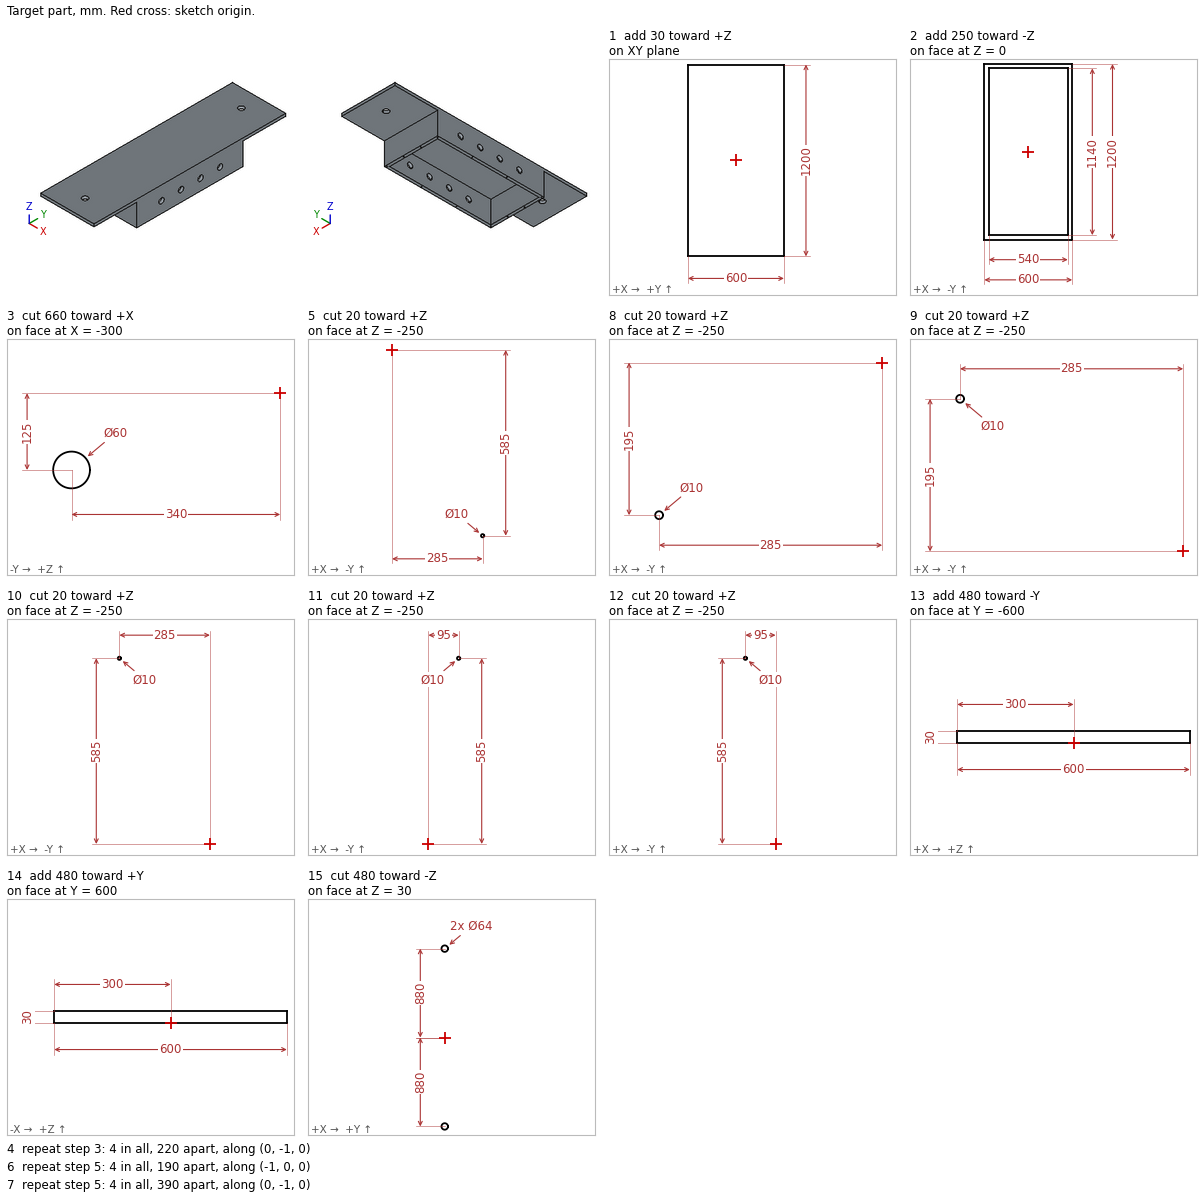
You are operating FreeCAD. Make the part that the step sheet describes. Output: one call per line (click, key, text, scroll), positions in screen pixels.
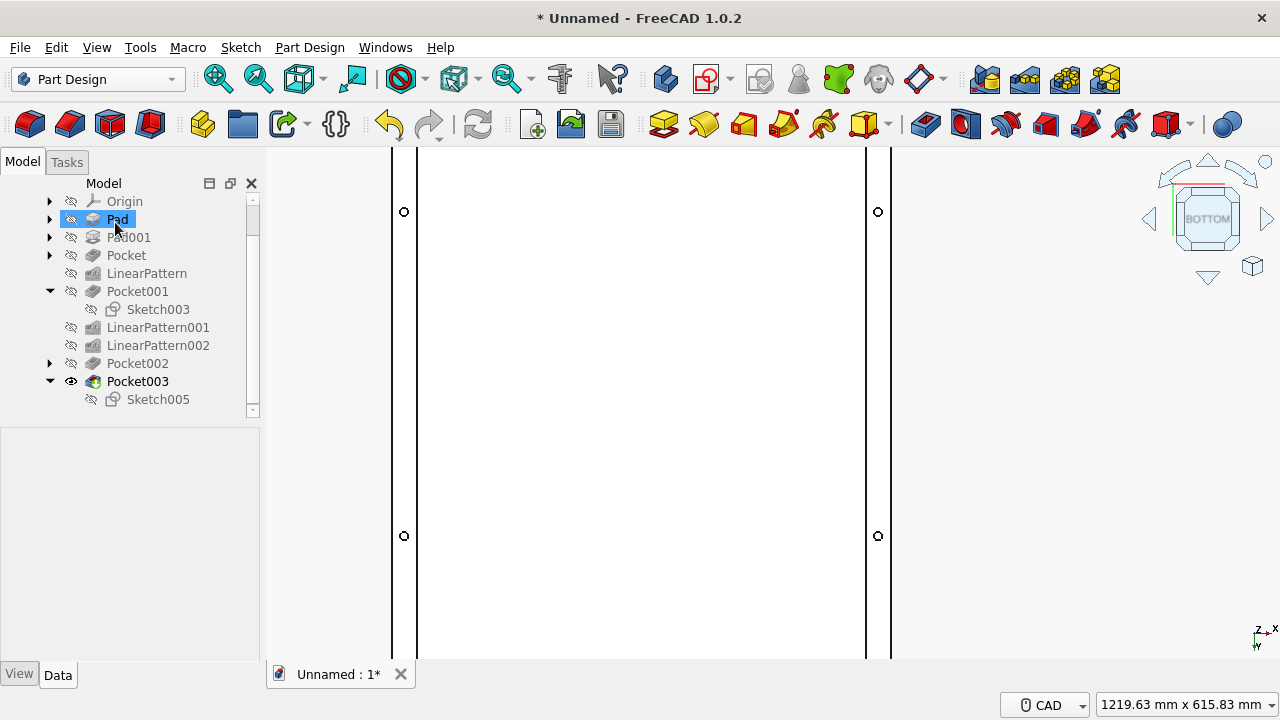
click(220, 80)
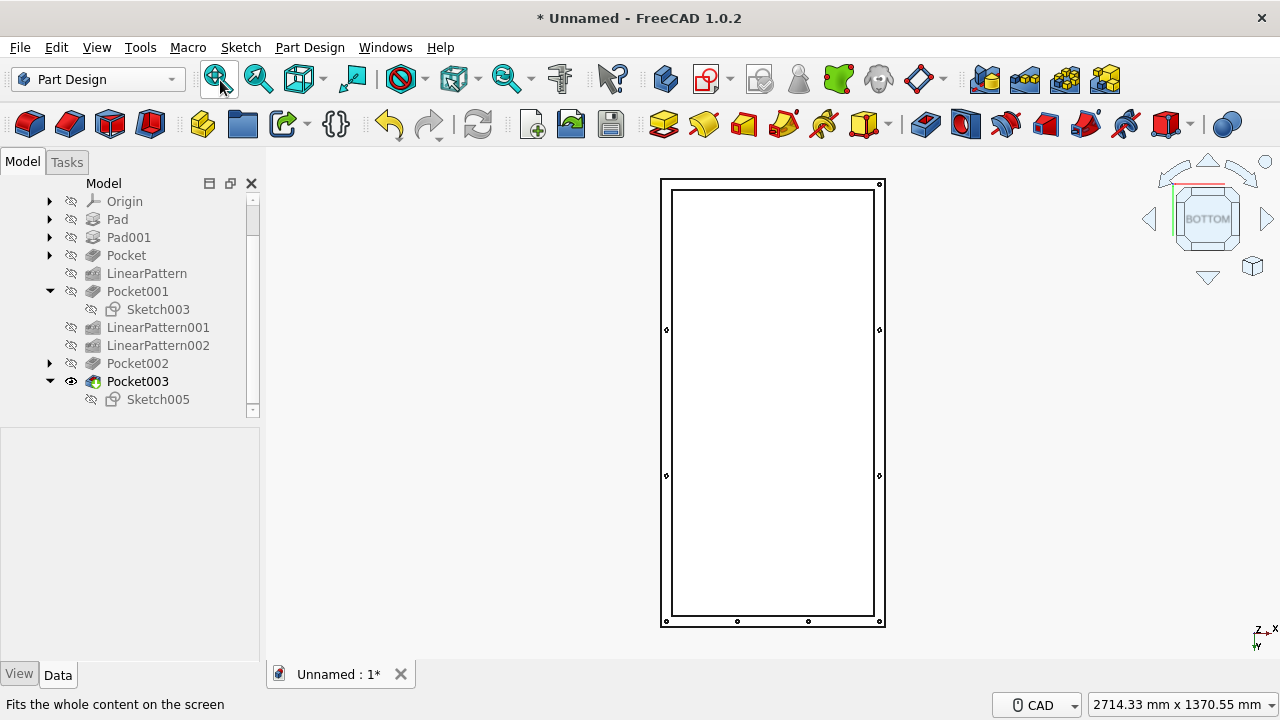
scroll(784, 621, up, 4)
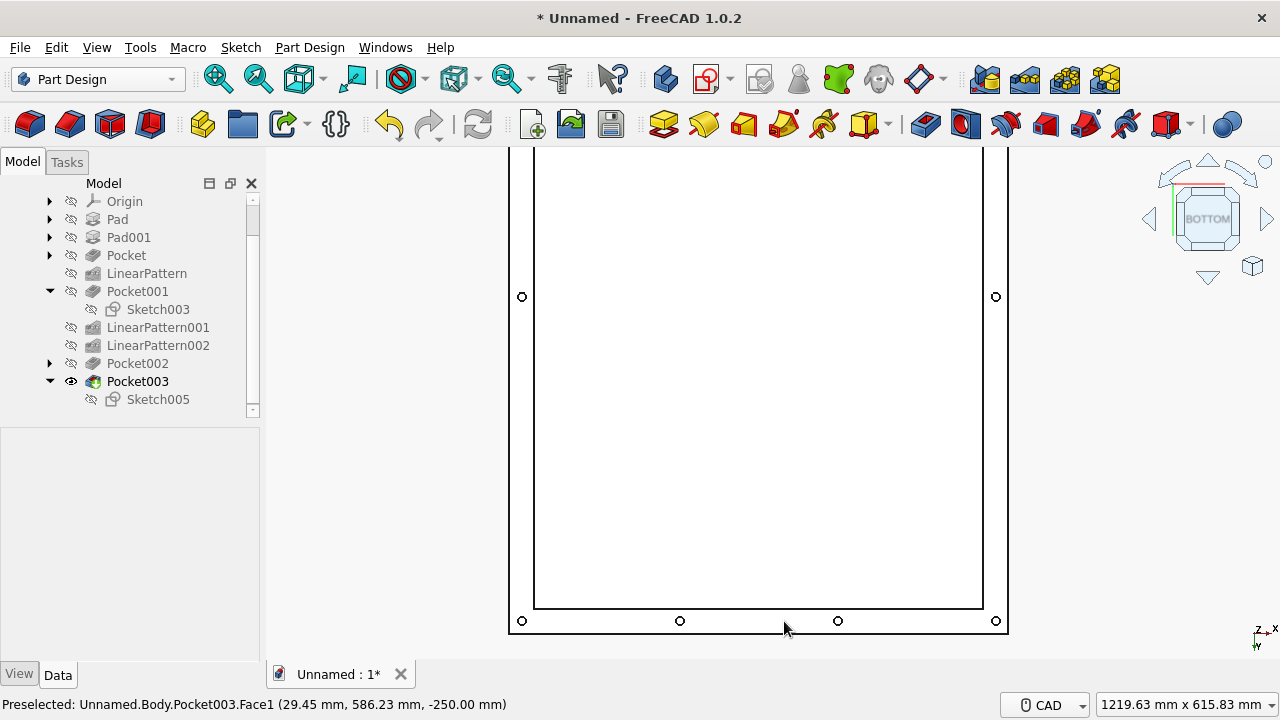
click(784, 620)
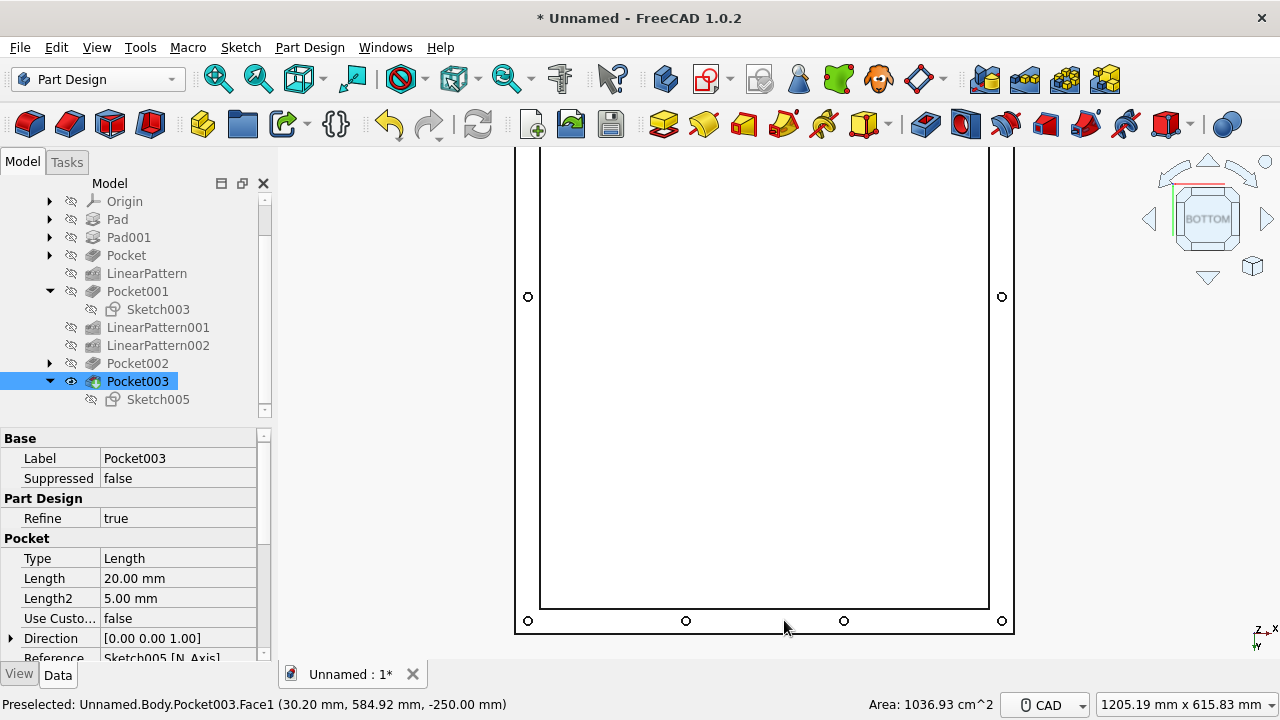
click(706, 80)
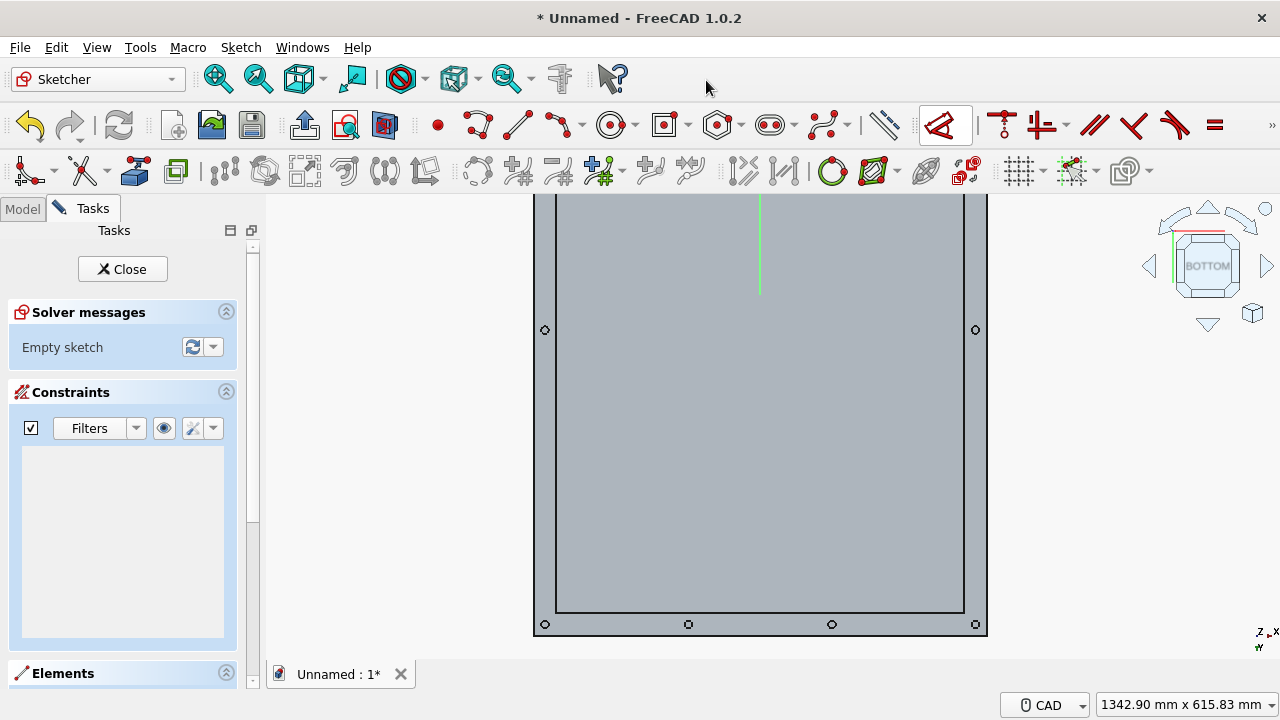
scroll(704, 426, down, 5)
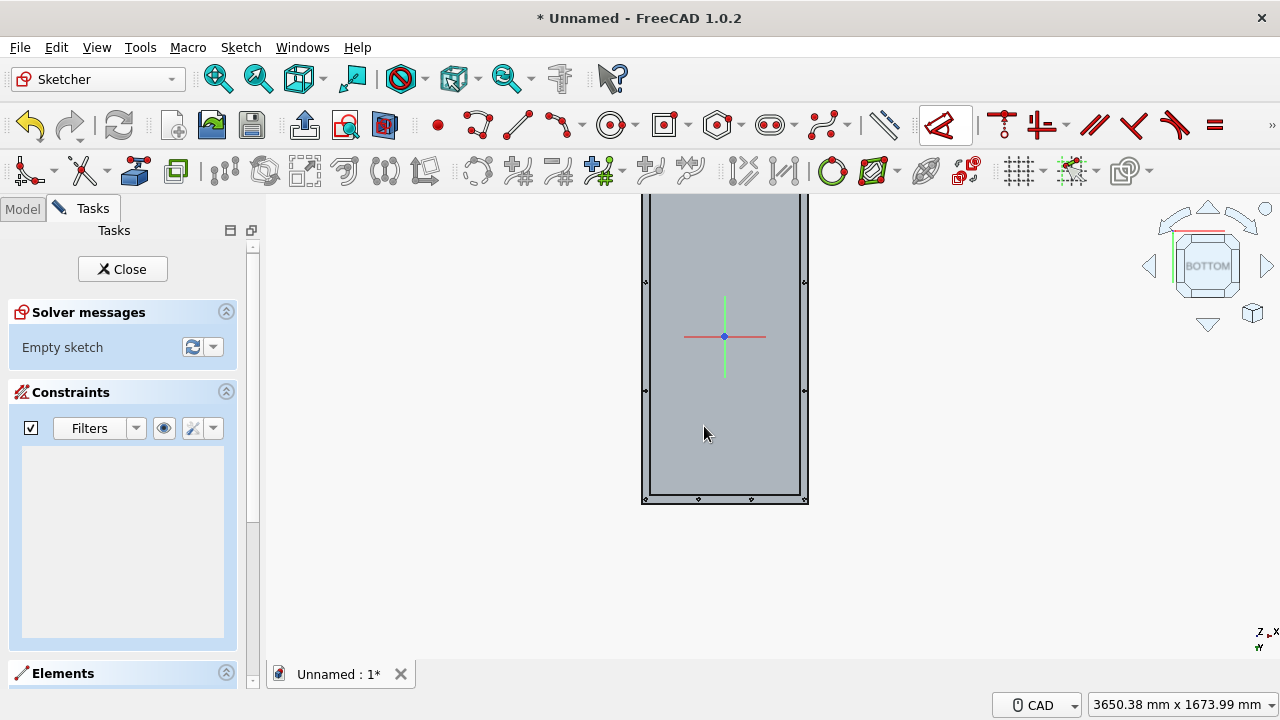
scroll(704, 426, down, 5)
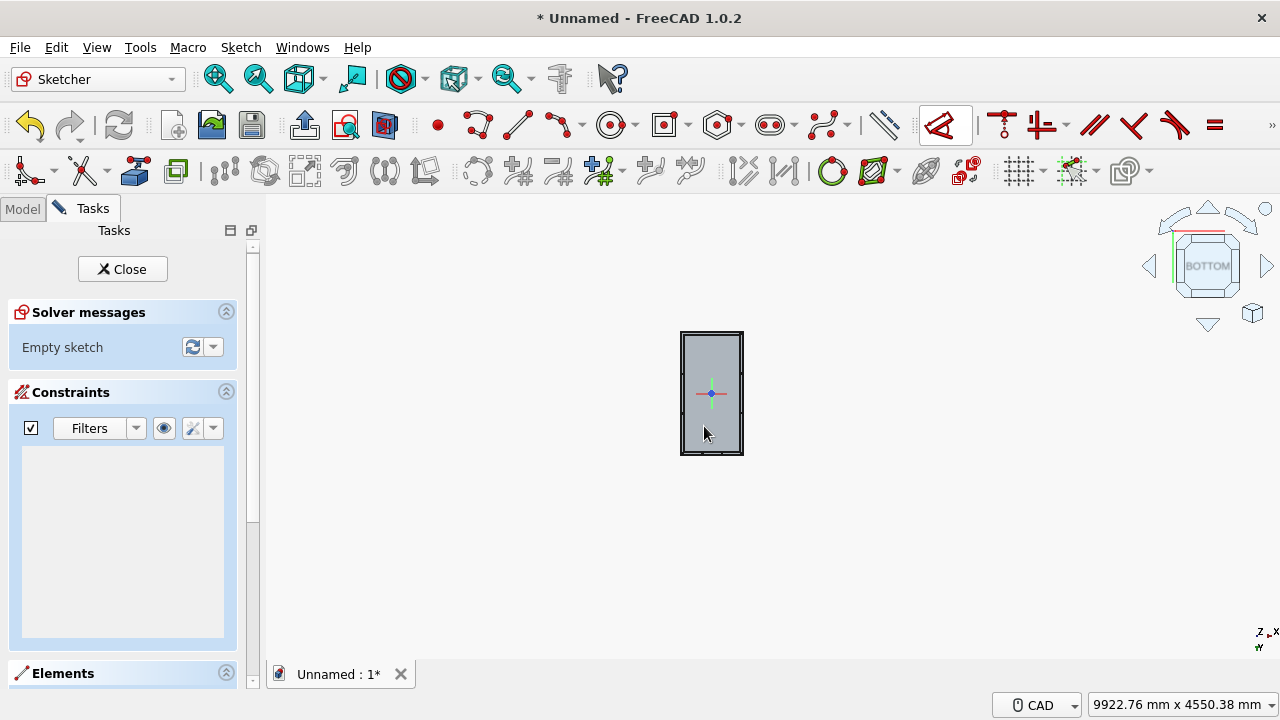
scroll(682, 329, up, 15)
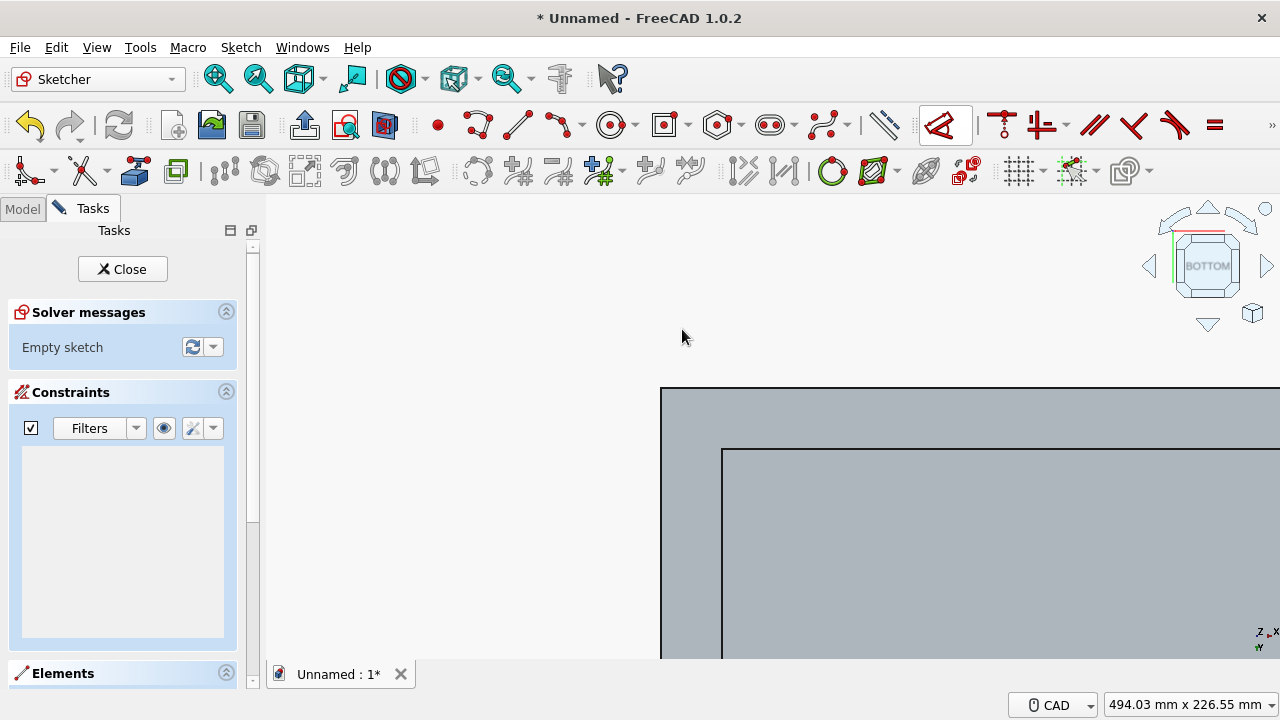
scroll(690, 418, up, 13)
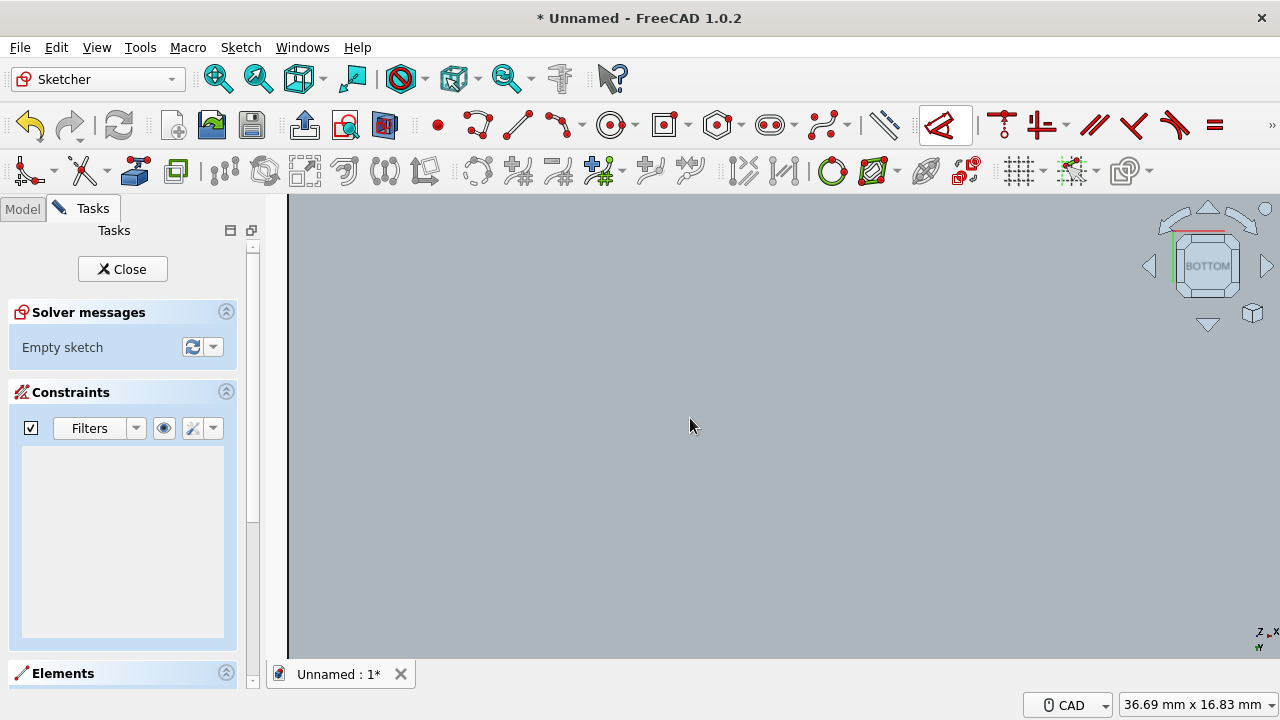
click(612, 126)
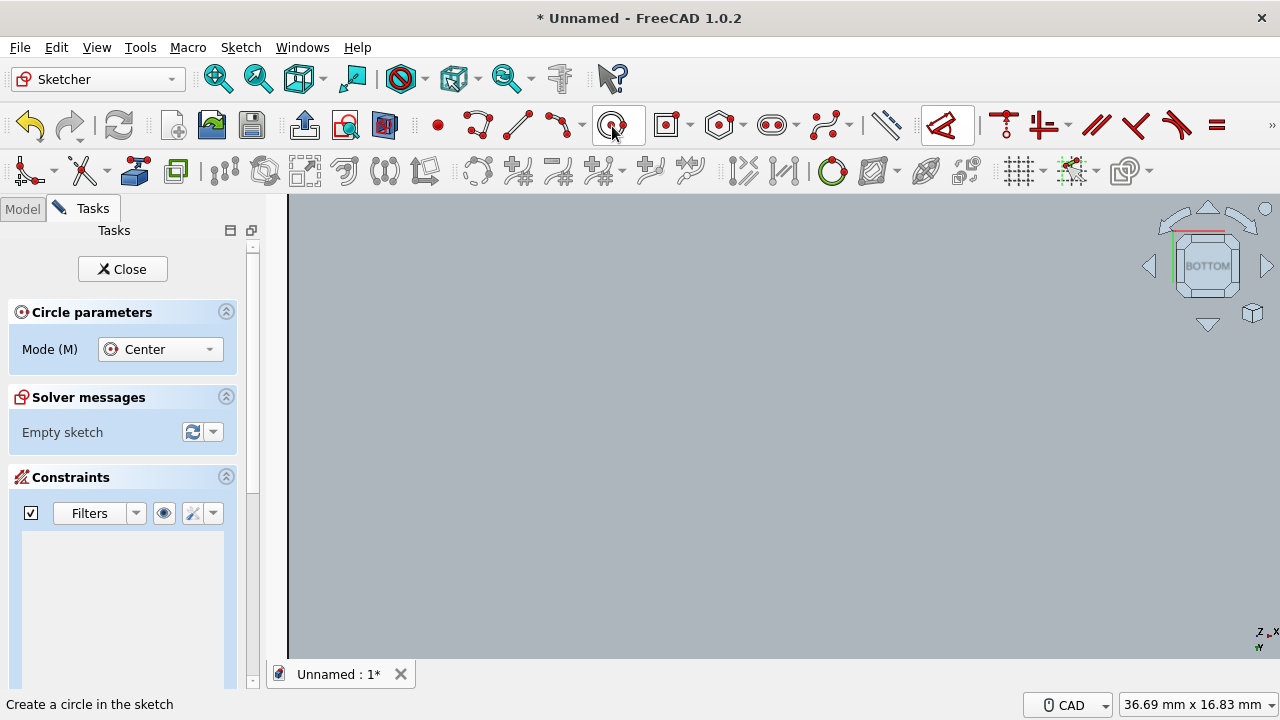
click(703, 421)
move(800, 323)